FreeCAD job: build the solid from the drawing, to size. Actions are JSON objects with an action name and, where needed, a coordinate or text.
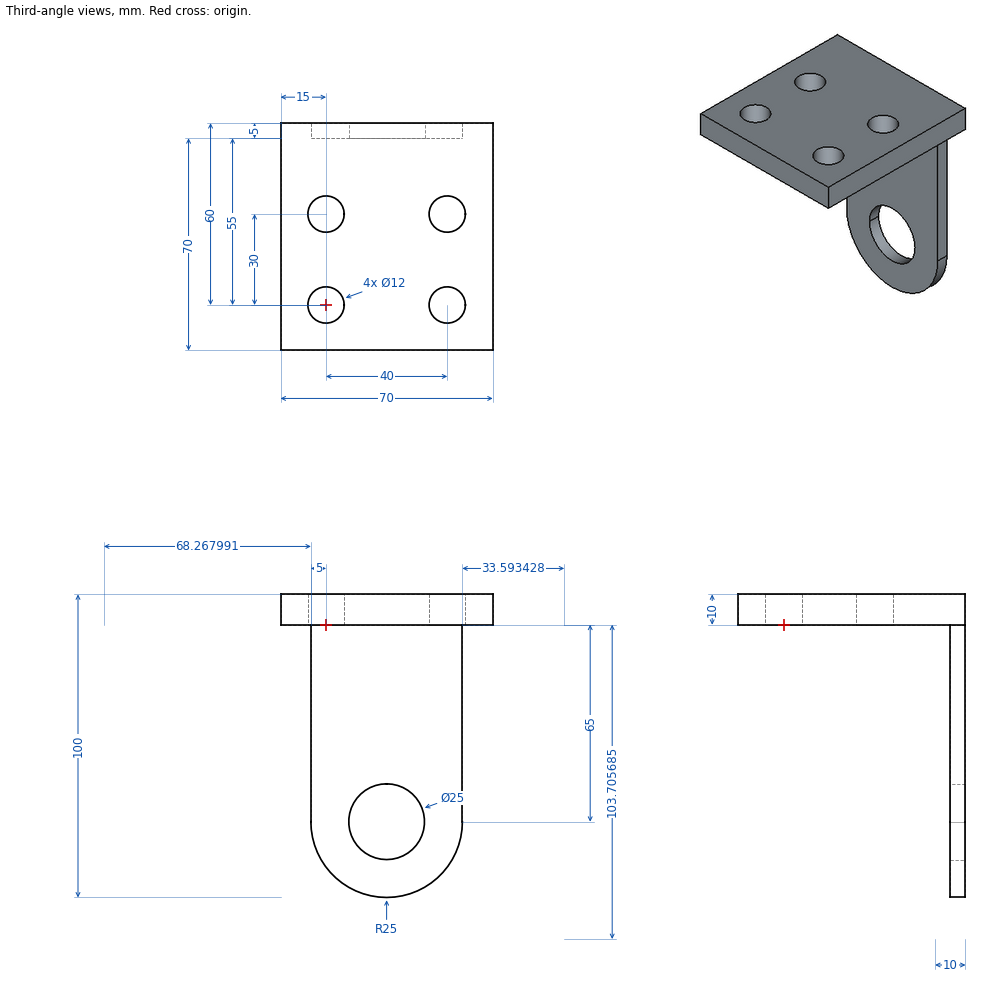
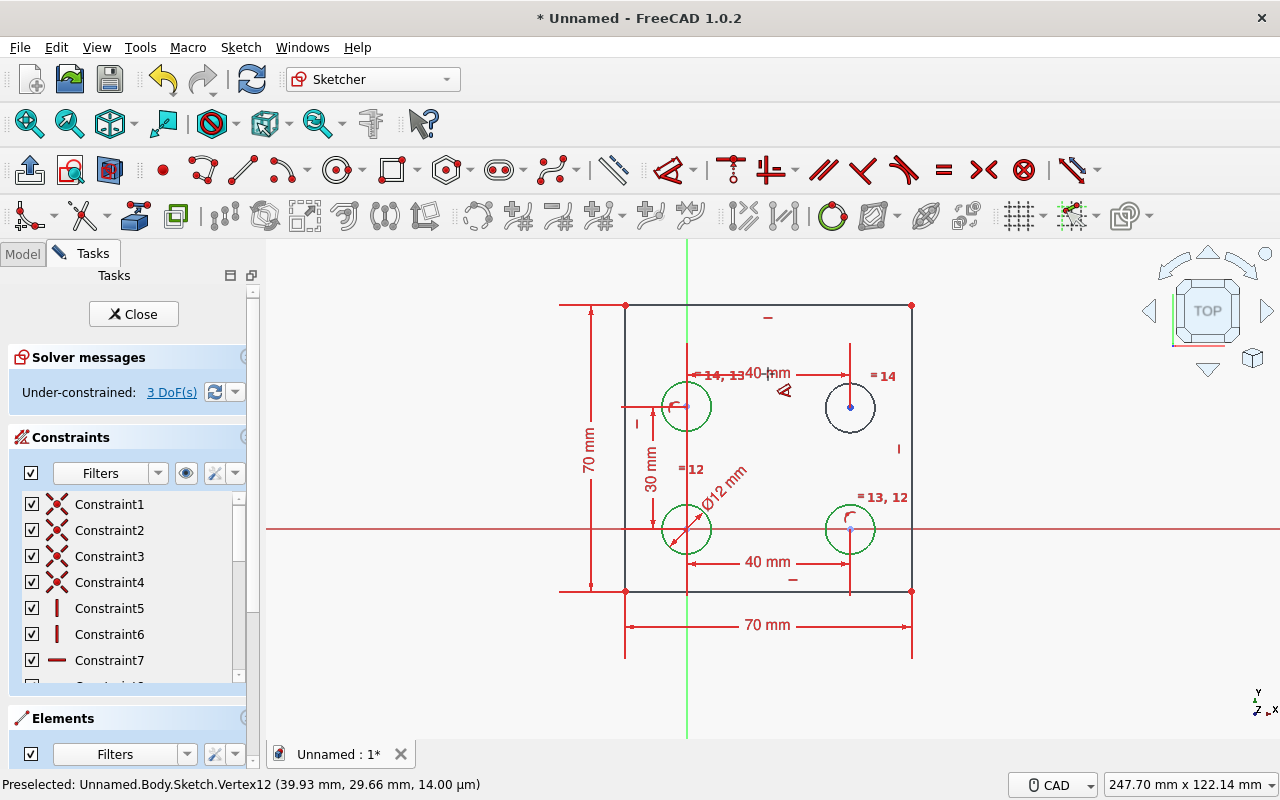
{"action": "left_click", "coordinate": [850, 408]}
{"action": "left_click", "coordinate": [884, 469]}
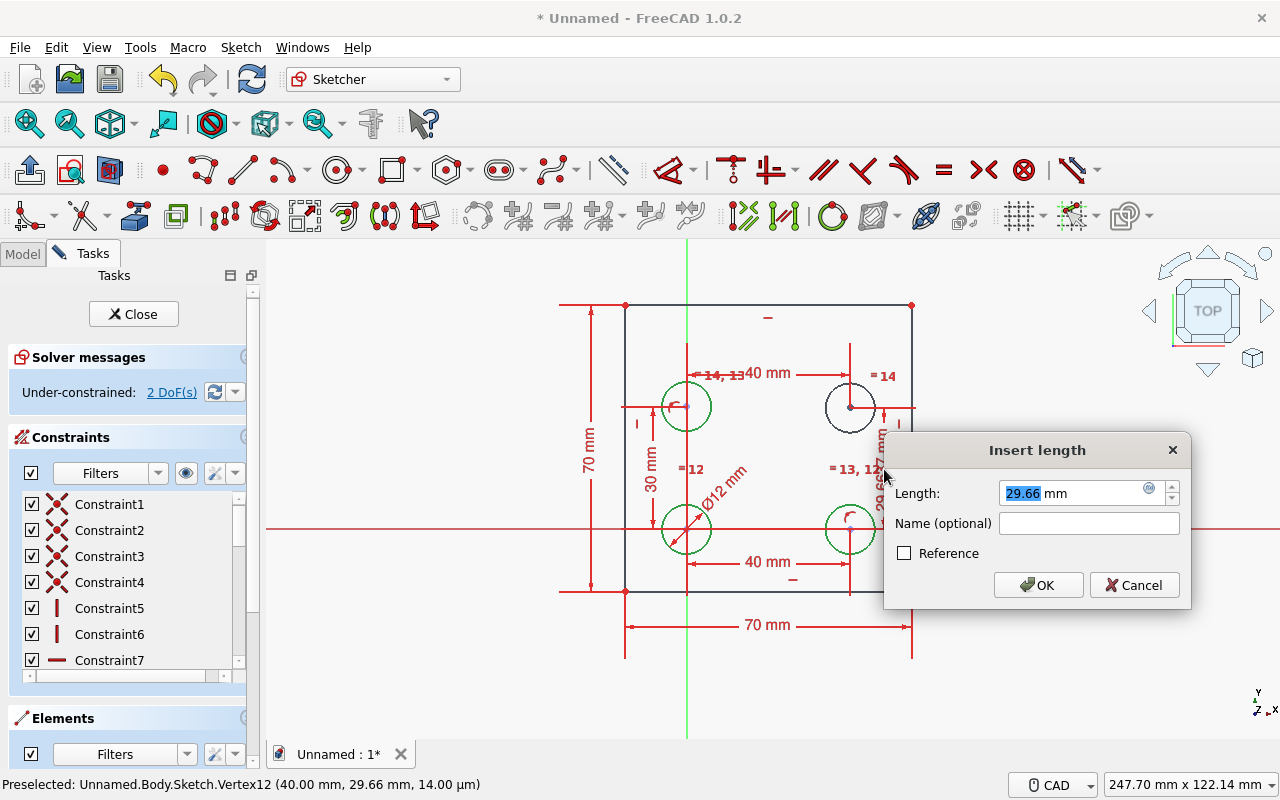
{"action": "type", "text": "30"}
{"action": "key", "text": "Return"}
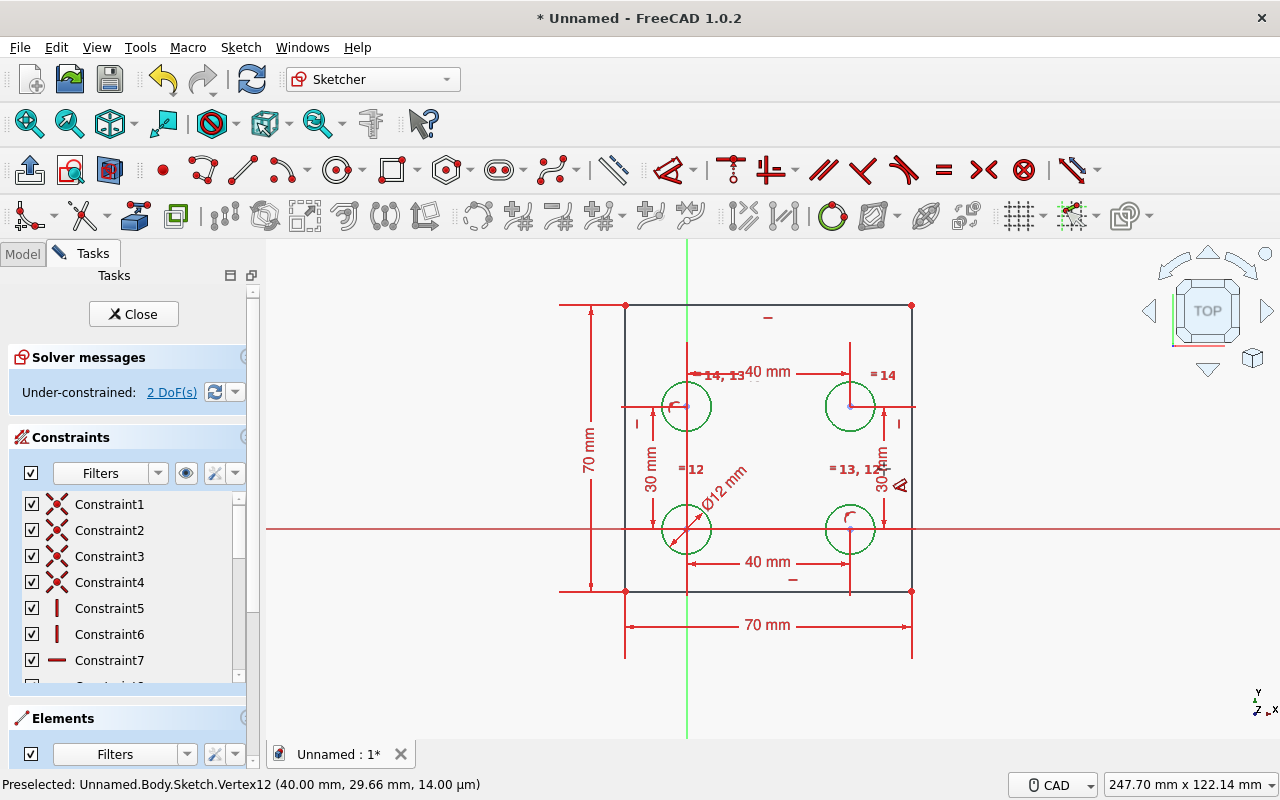
{"action": "left_click", "coordinate": [625, 305]}
{"action": "left_click", "coordinate": [656, 271]}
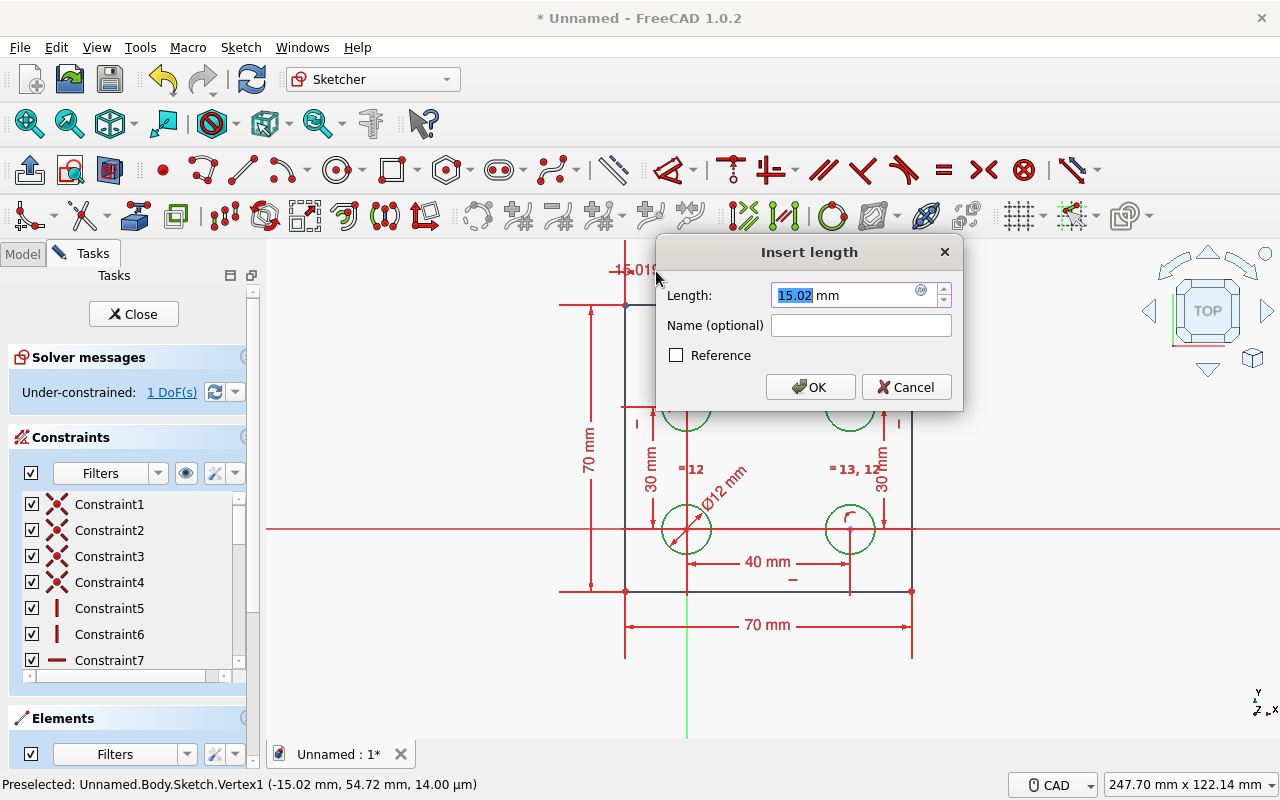
{"action": "type", "text": "15"}
{"action": "key", "text": "Return"}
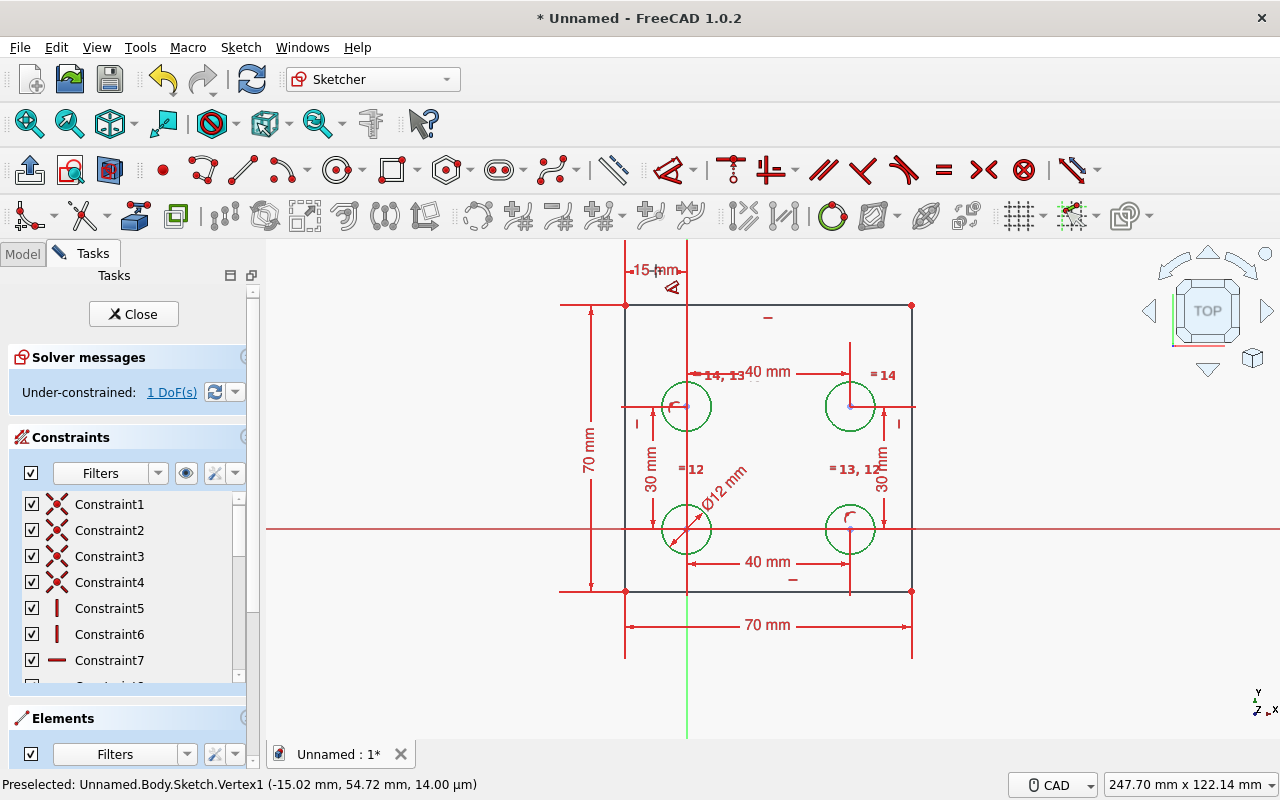
{"action": "left_click", "coordinate": [625, 305]}
{"action": "left_click", "coordinate": [591, 417]}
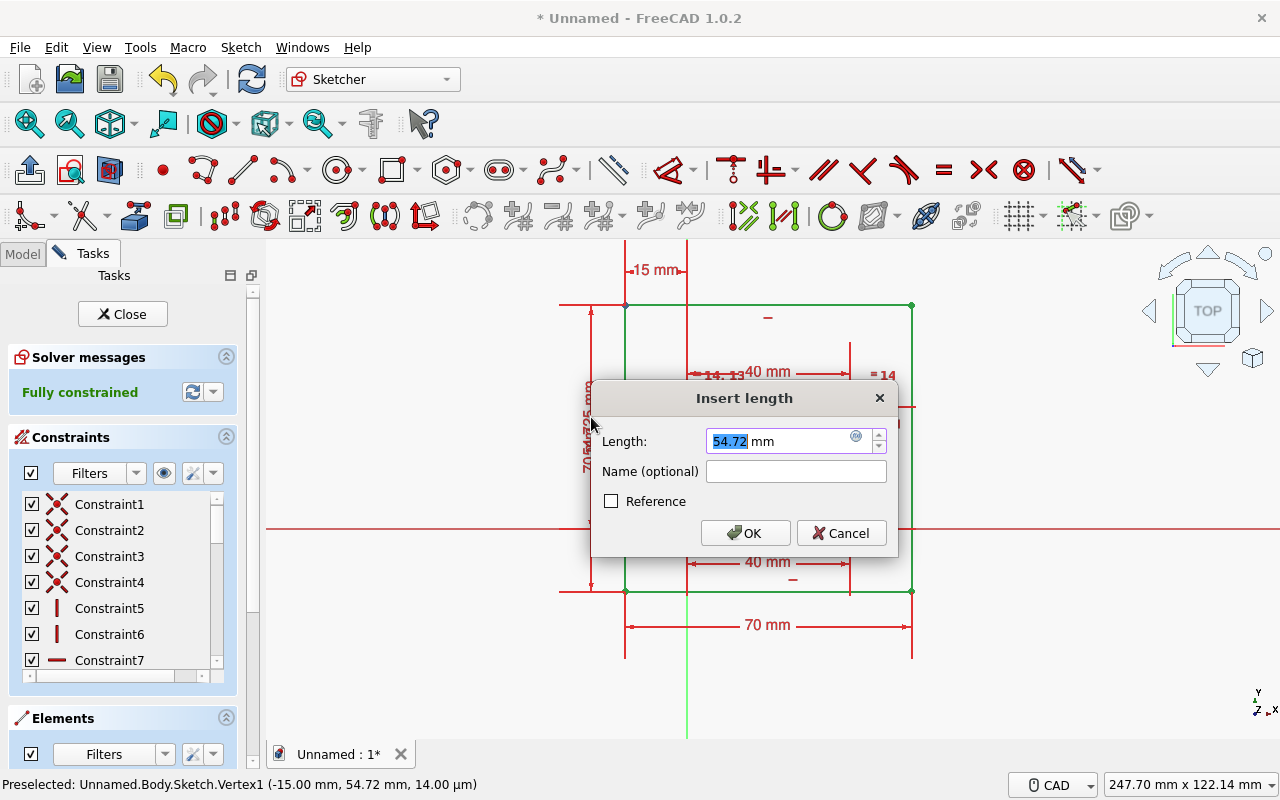
{"action": "type", "text": "55"}
{"action": "key", "text": "Return"}
{"action": "key", "text": "Escape"}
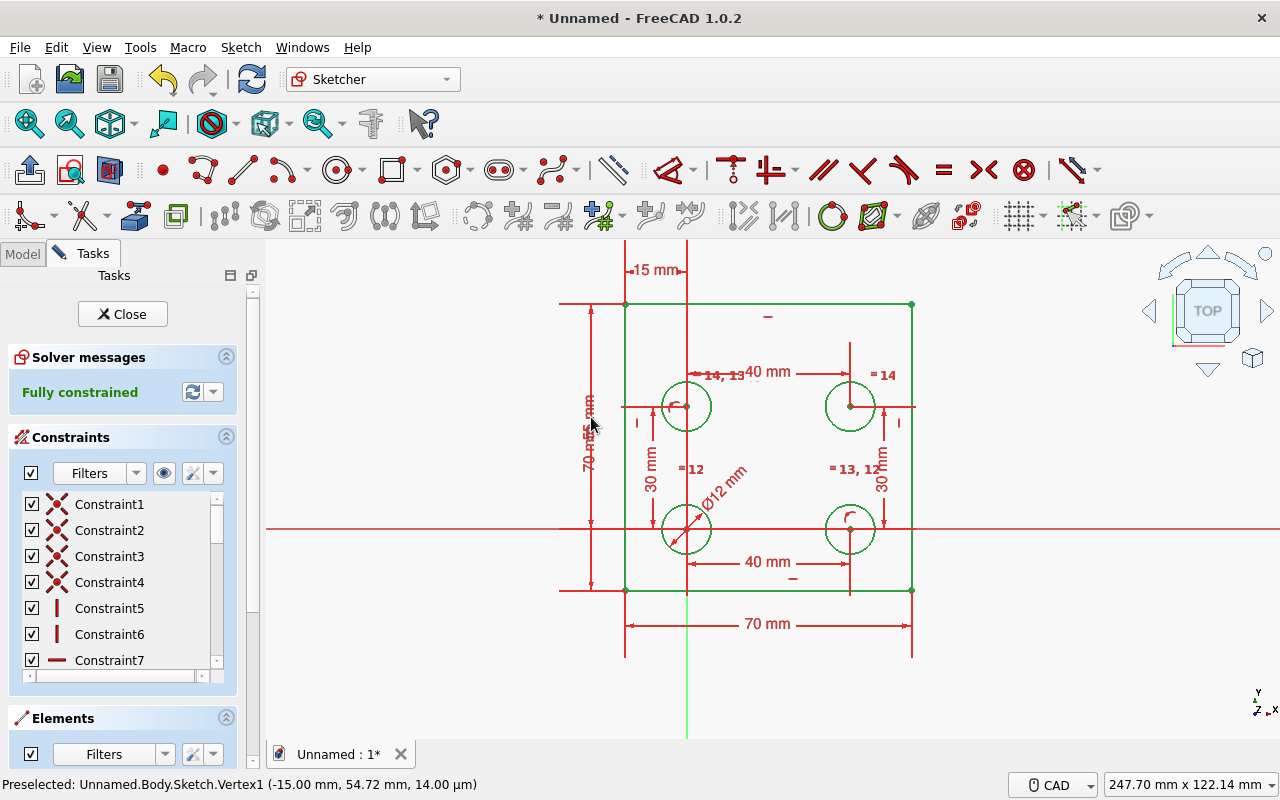
{"action": "left_click", "coordinate": [123, 314]}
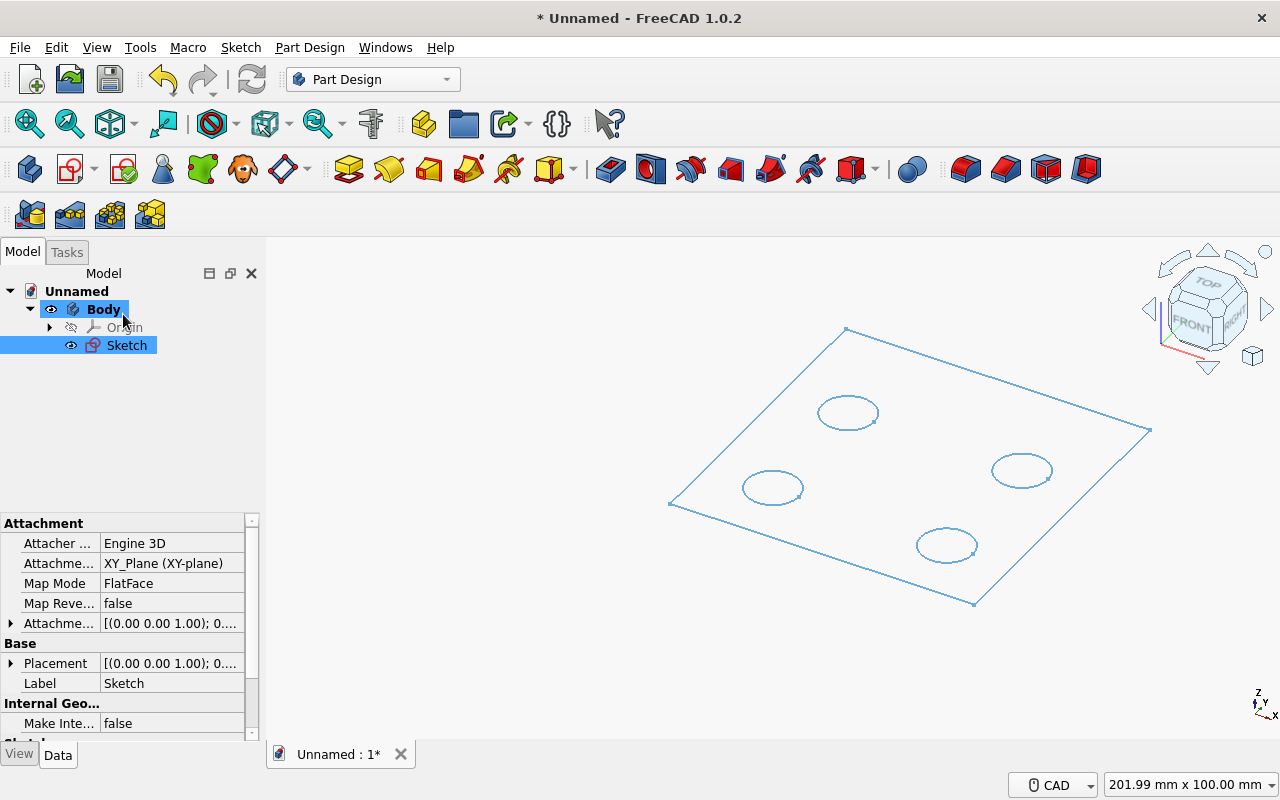
{"action": "left_click", "coordinate": [350, 170]}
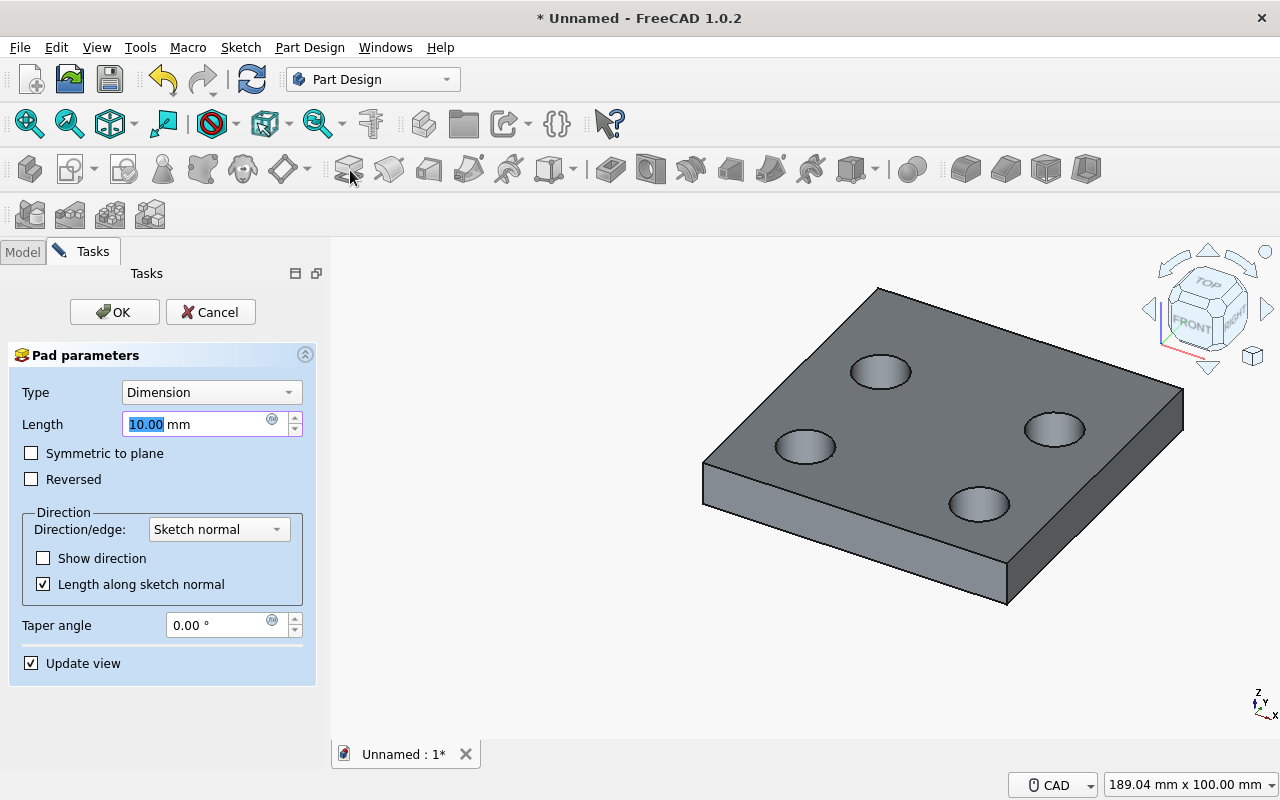
{"action": "type", "text": "10"}
{"action": "key", "text": "Tab"}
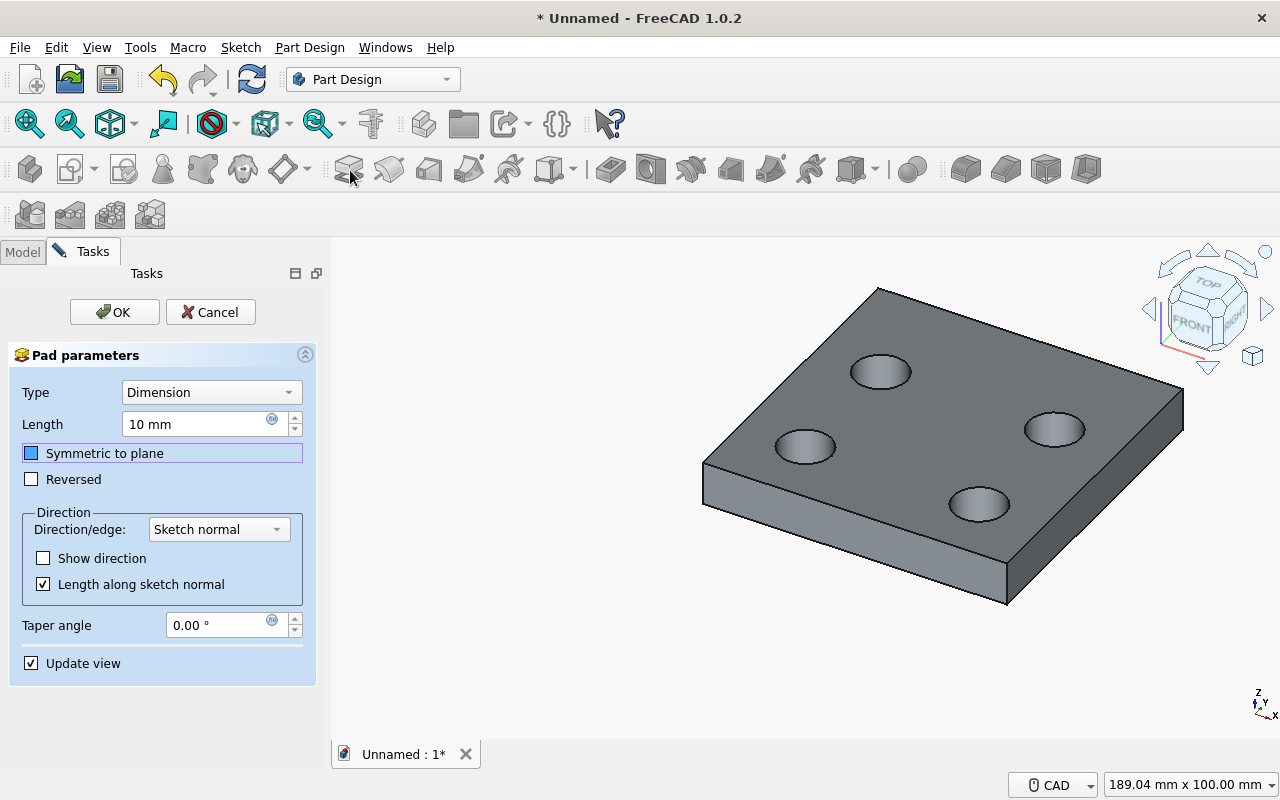
{"action": "left_click", "coordinate": [115, 312]}